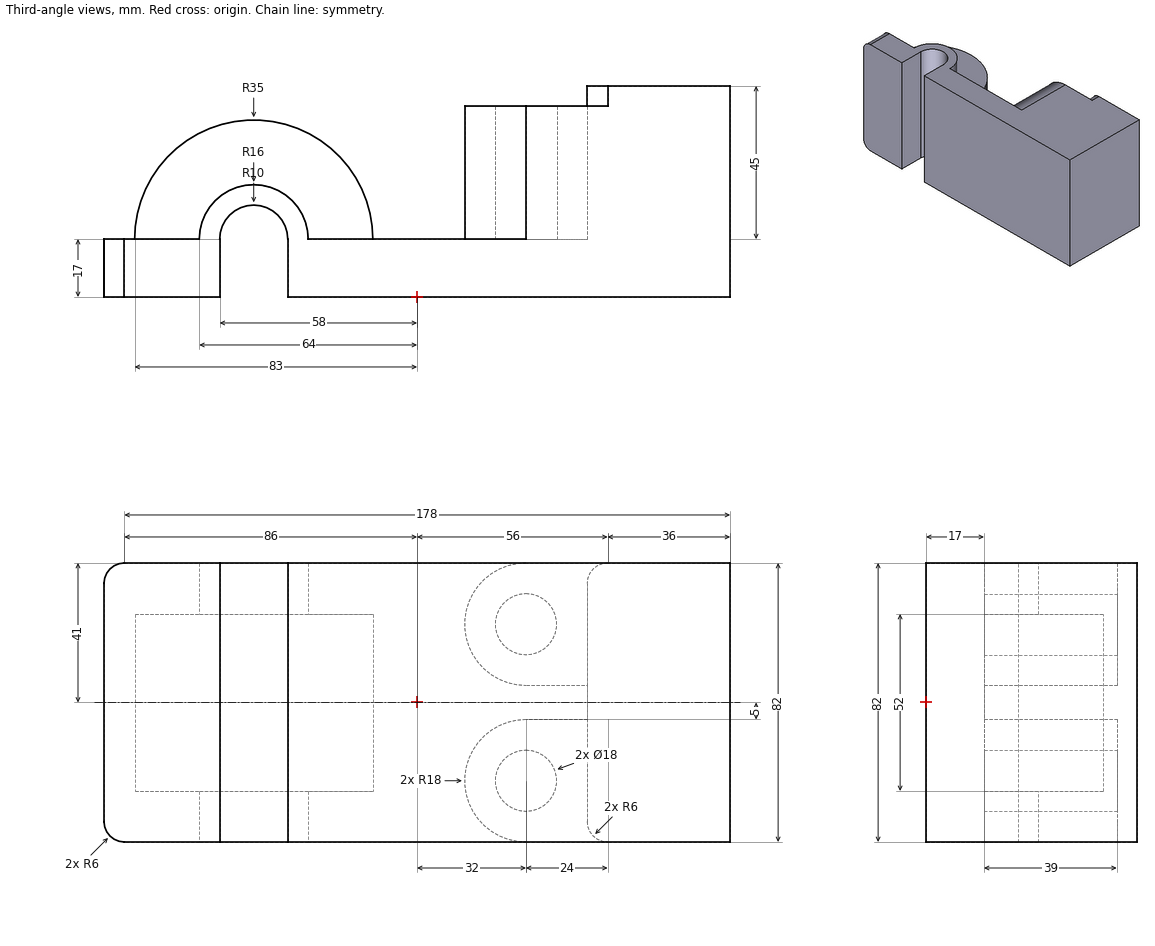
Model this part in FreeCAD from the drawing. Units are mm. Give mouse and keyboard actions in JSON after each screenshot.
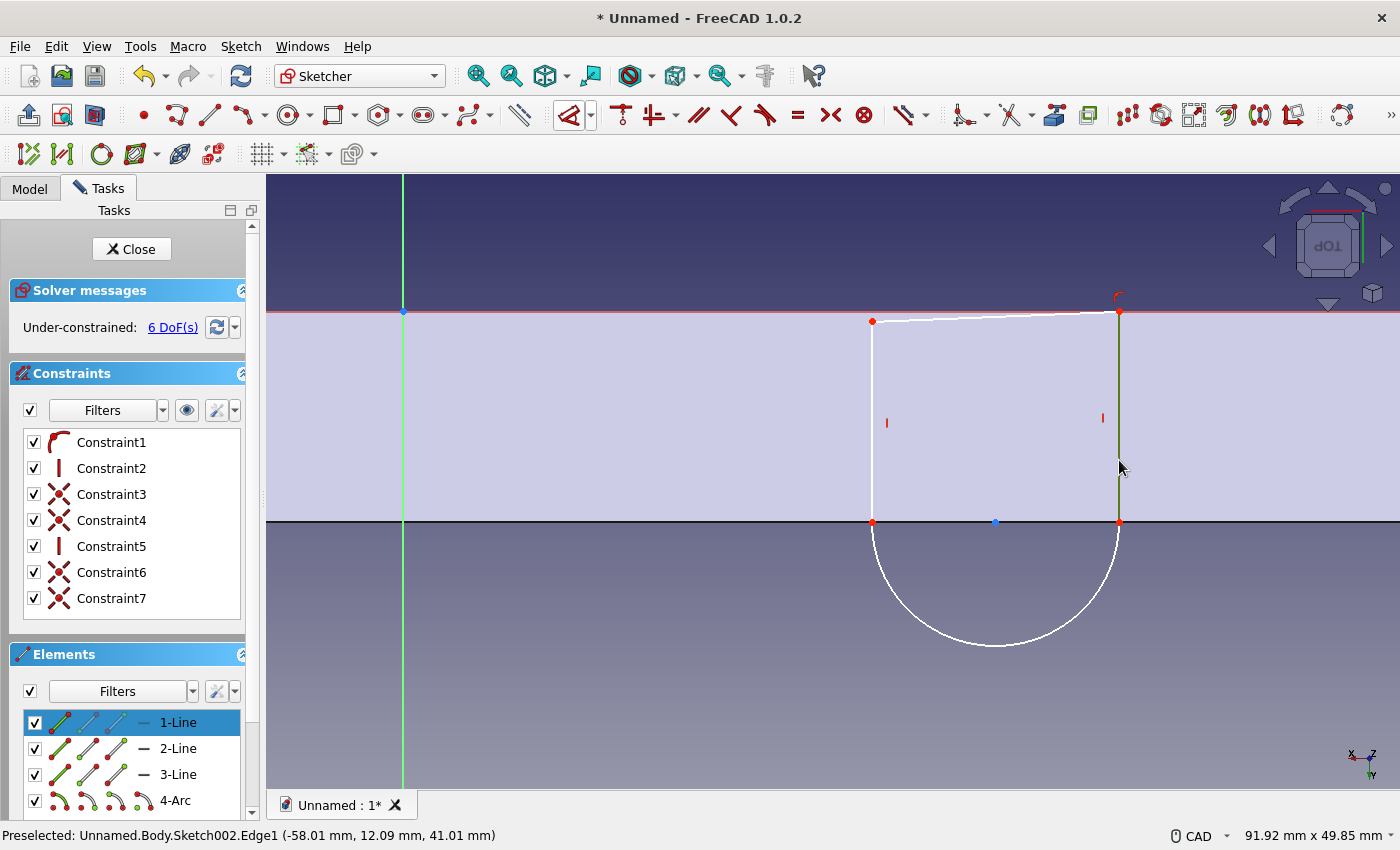
{"action": "left_click", "coordinate": [923, 623]}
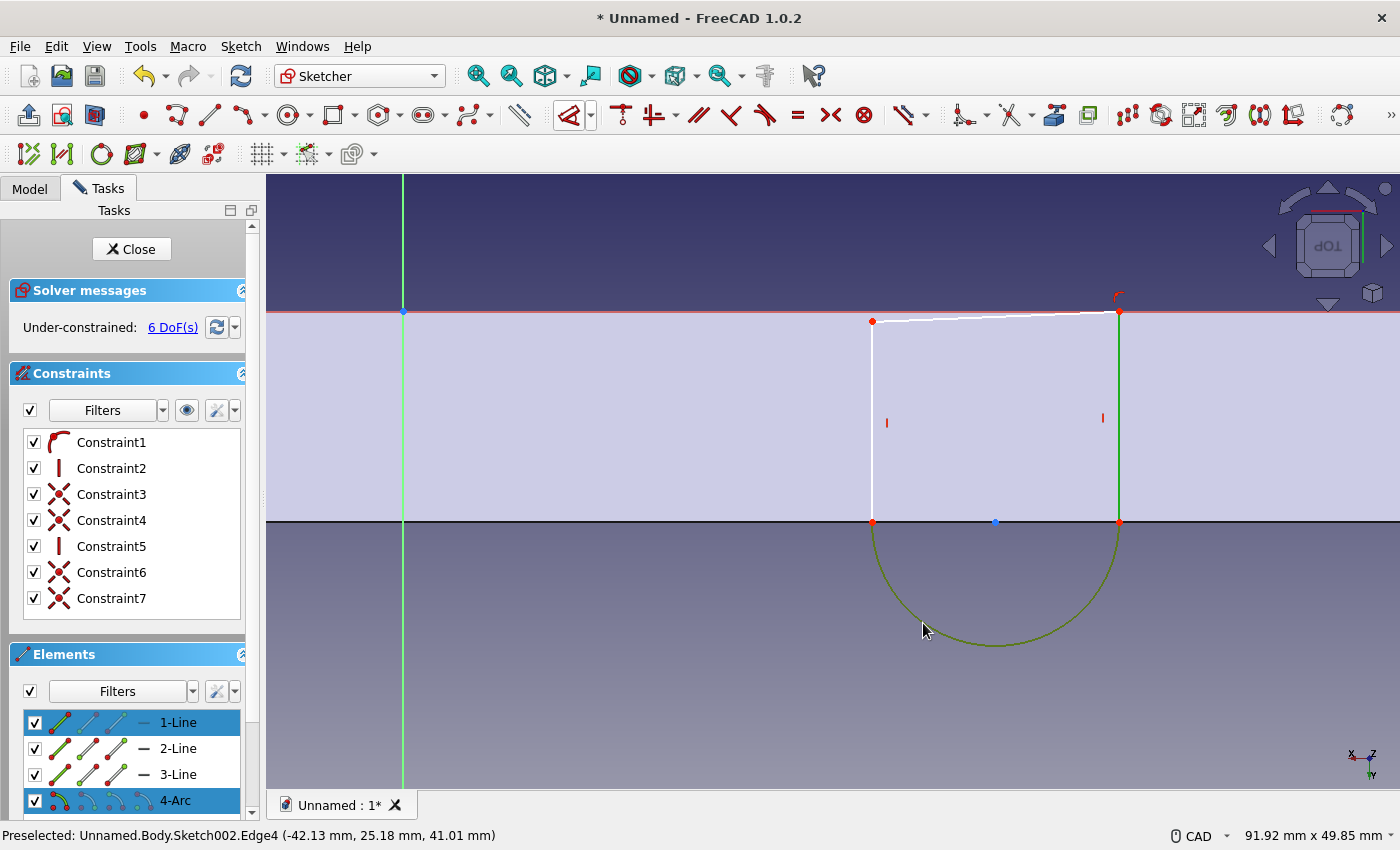
{"action": "left_click", "coordinate": [765, 116]}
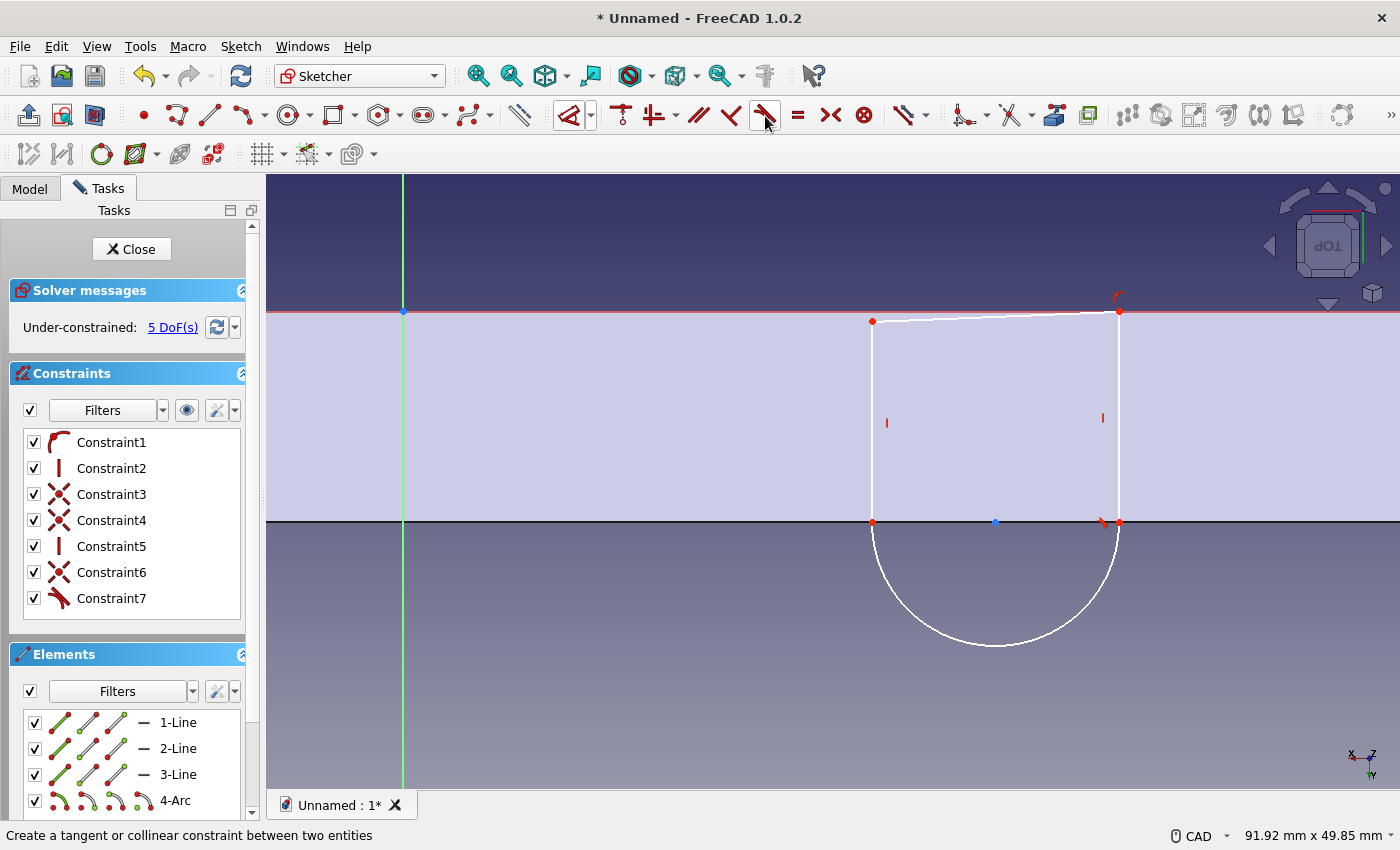
{"action": "left_click", "coordinate": [872, 382]}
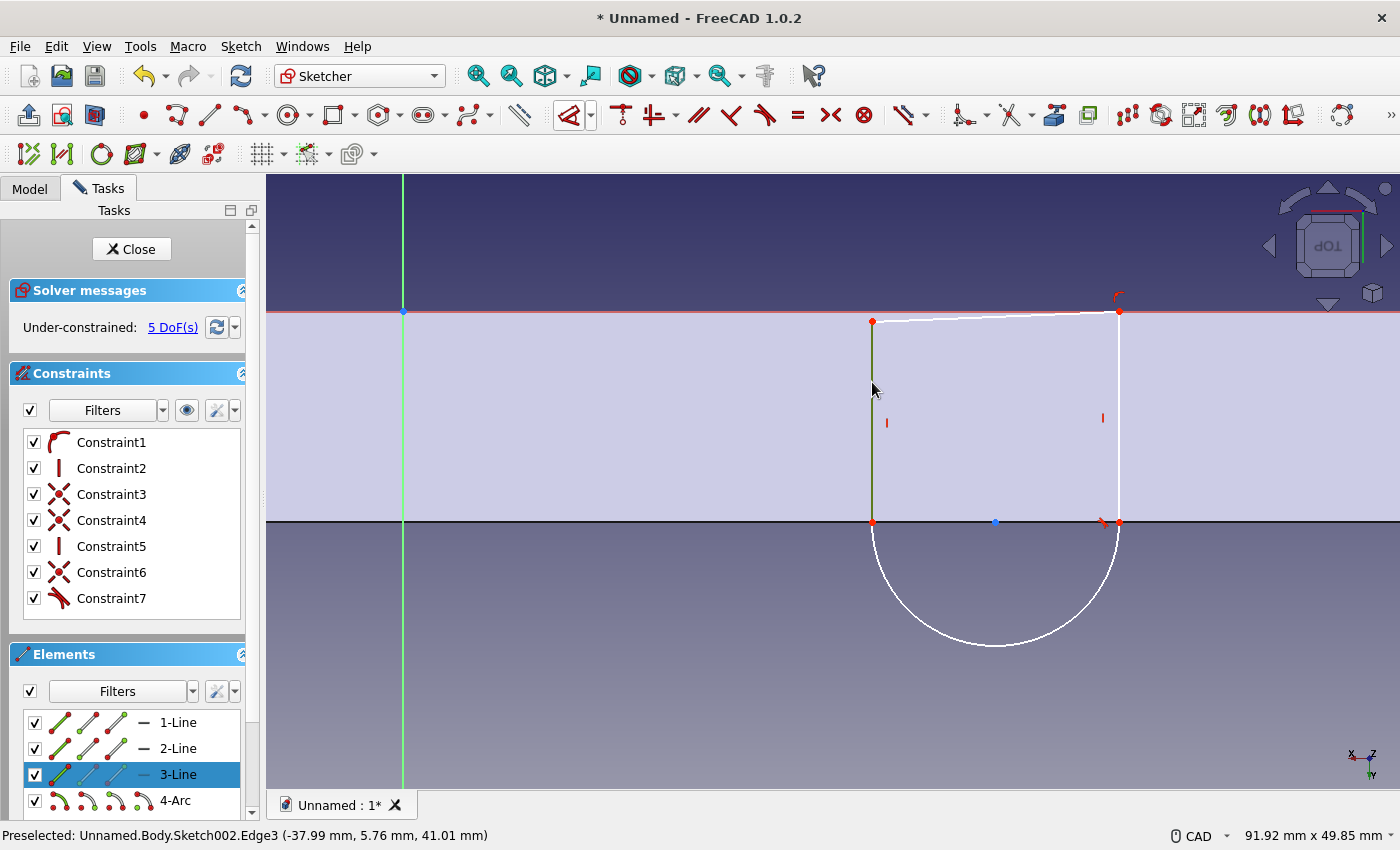
{"action": "left_click", "coordinate": [923, 623]}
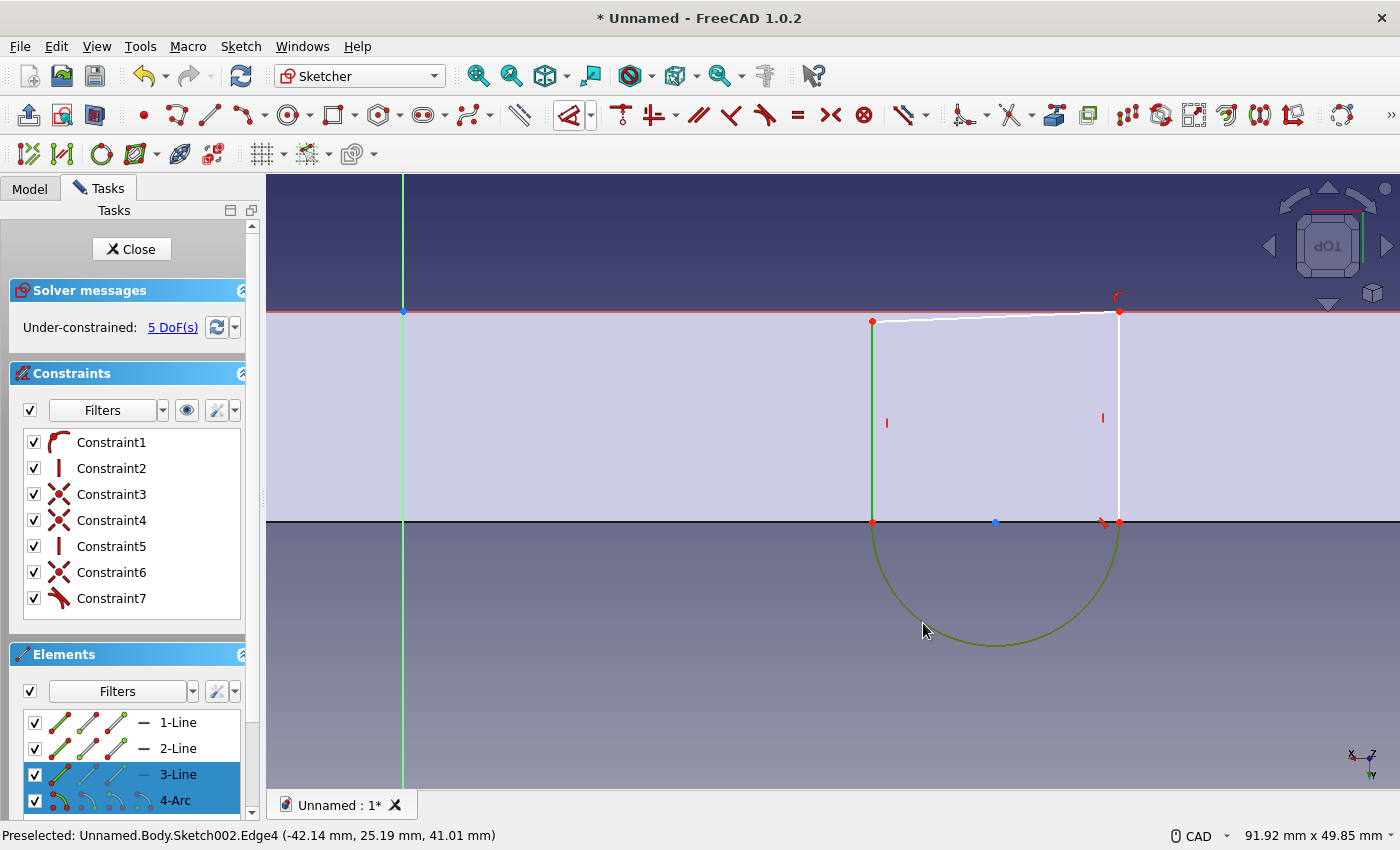
{"action": "left_click", "coordinate": [765, 116]}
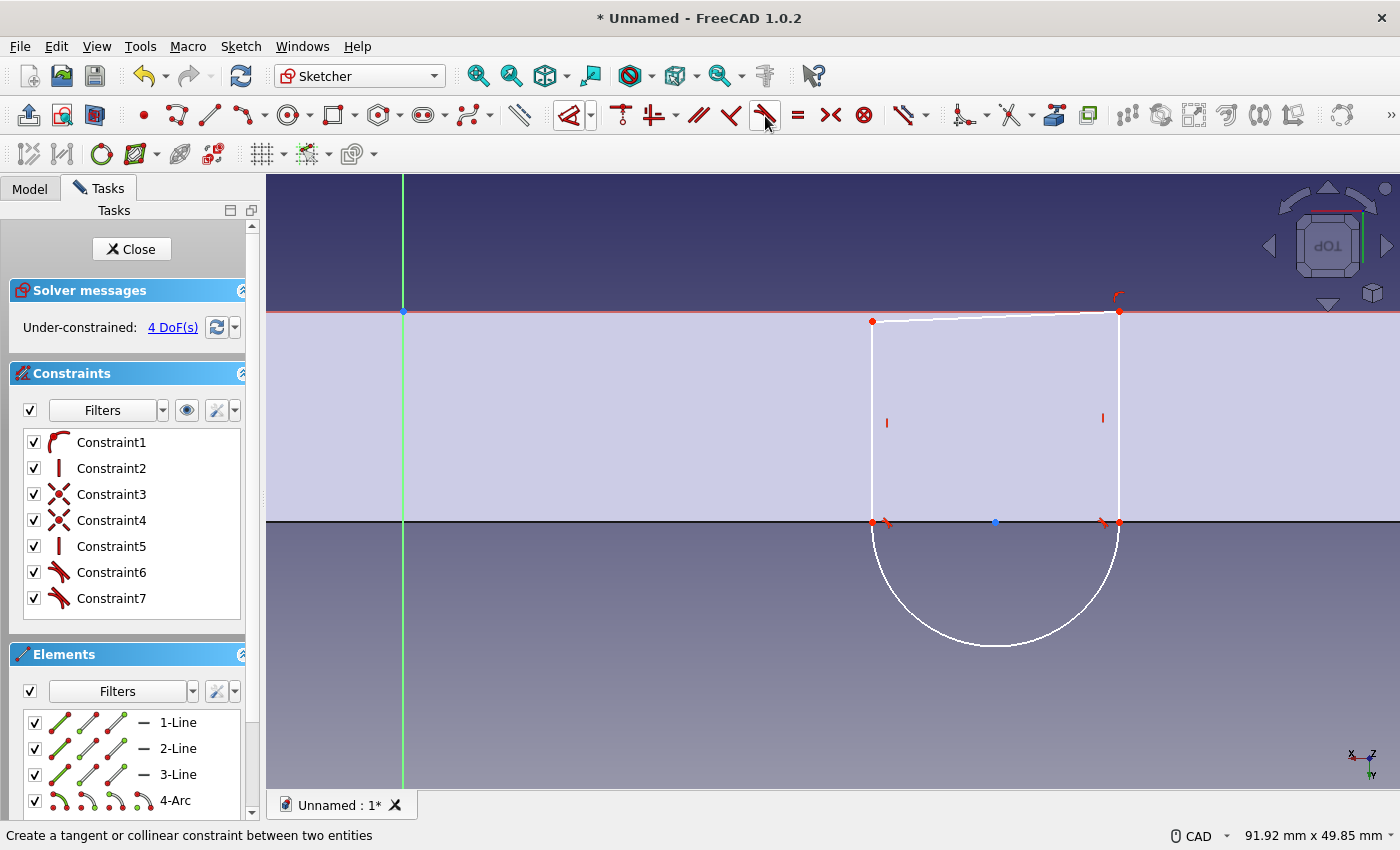
{"action": "left_click", "coordinate": [1045, 315]}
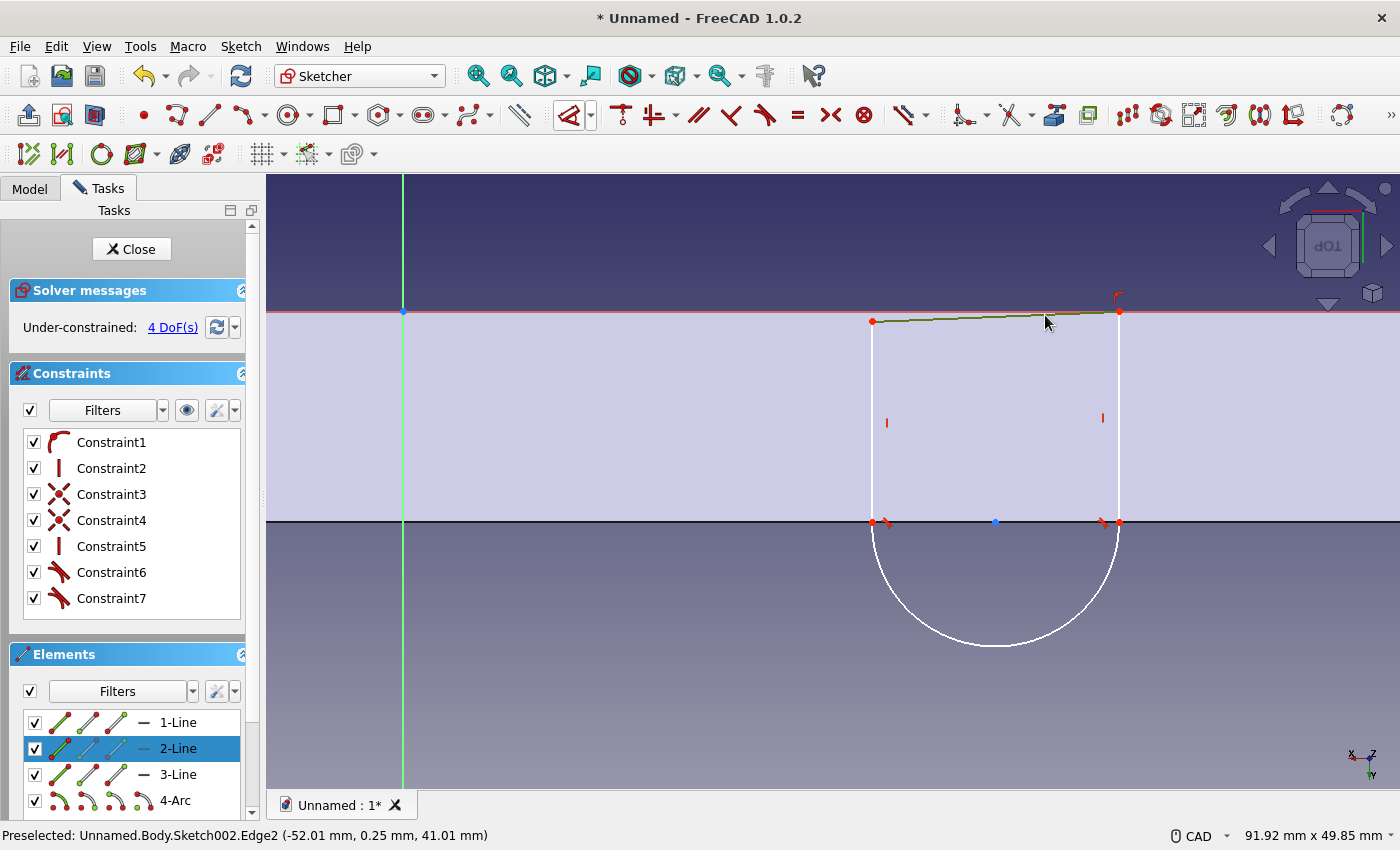
{"action": "left_click", "coordinate": [676, 116]}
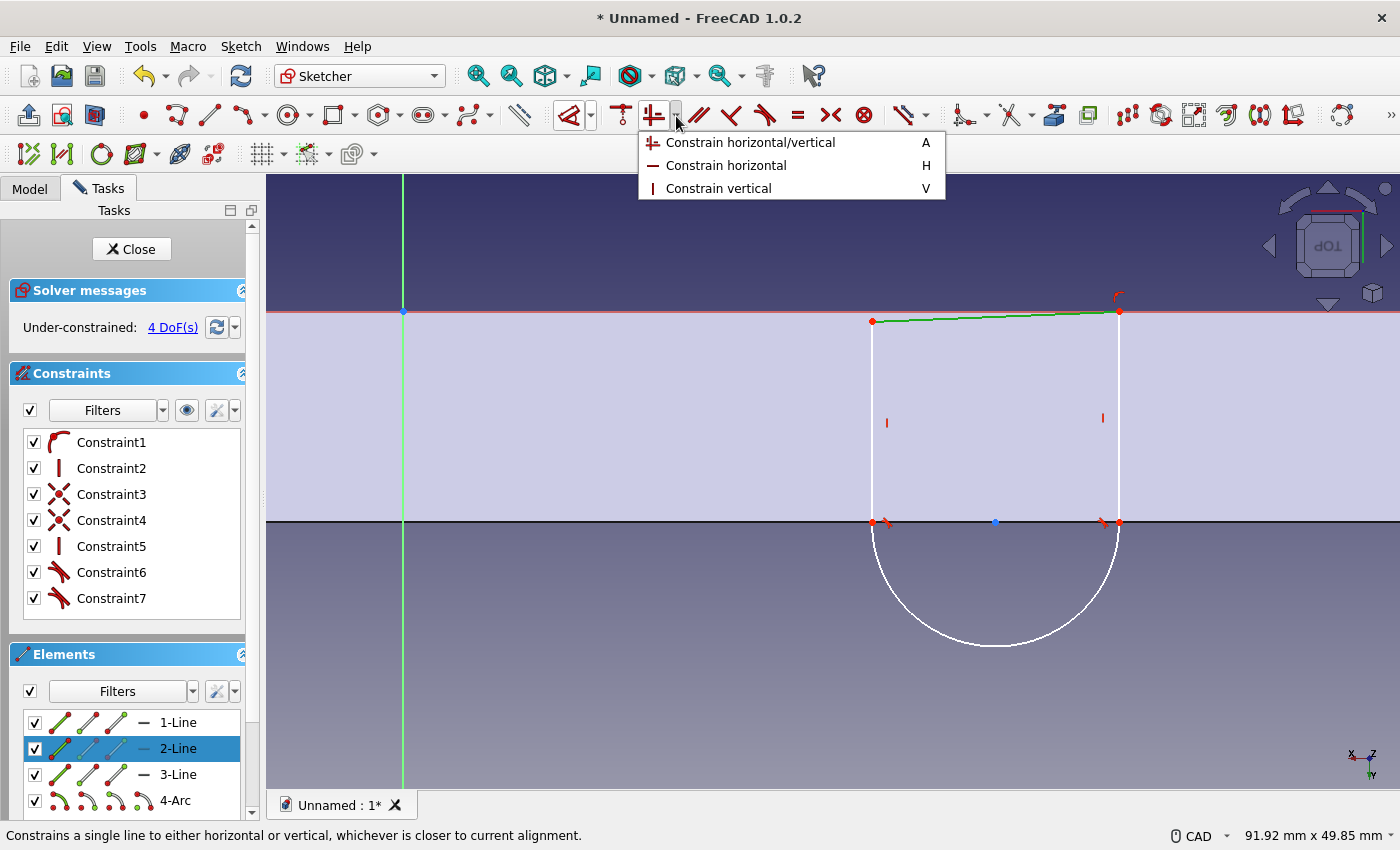
{"action": "left_click", "coordinate": [792, 166]}